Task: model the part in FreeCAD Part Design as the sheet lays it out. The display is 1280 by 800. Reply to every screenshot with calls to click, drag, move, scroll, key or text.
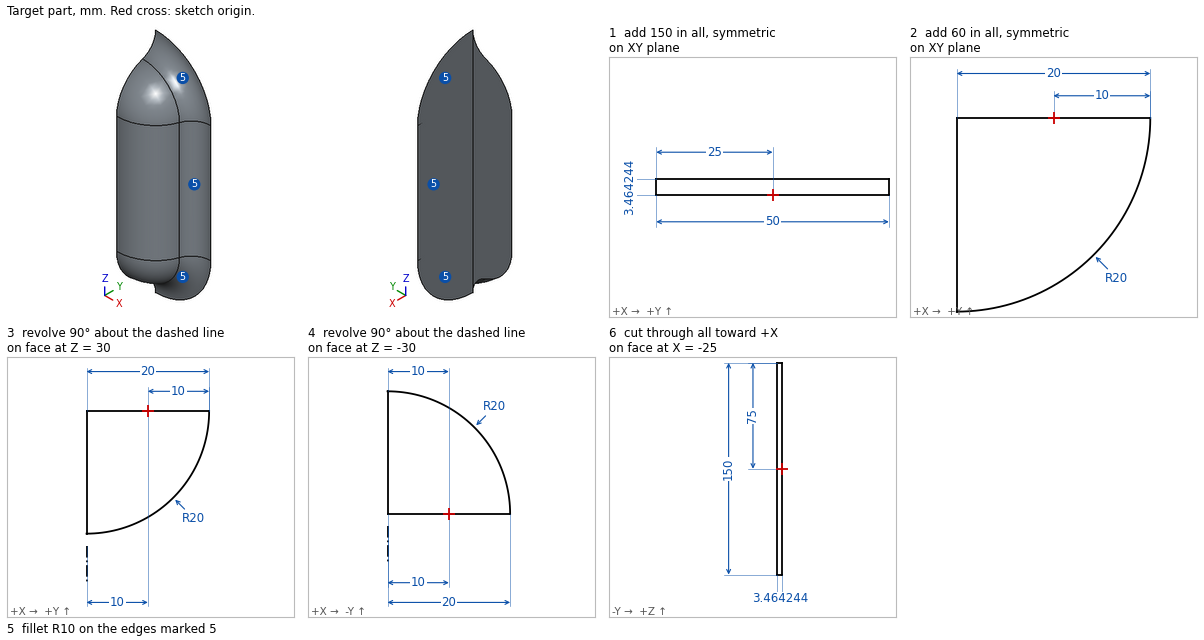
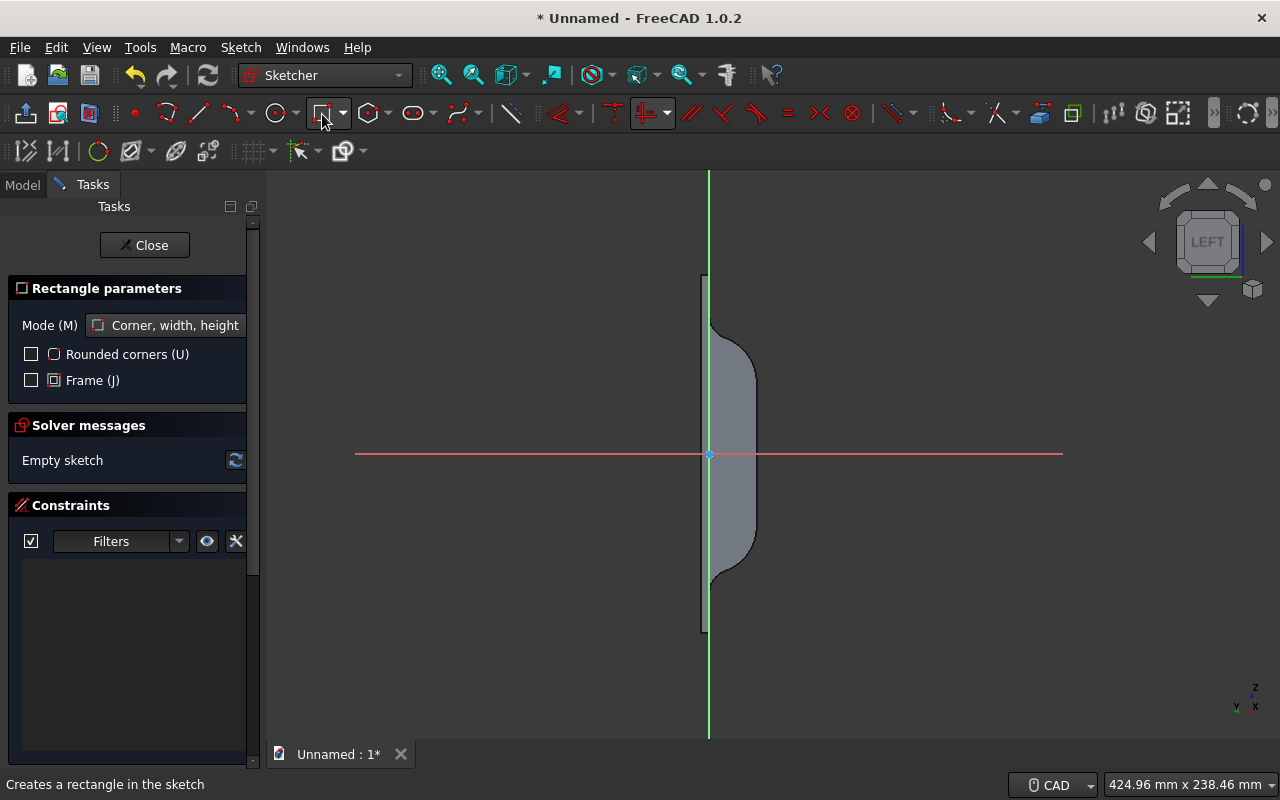
scroll(701, 275, up, 4)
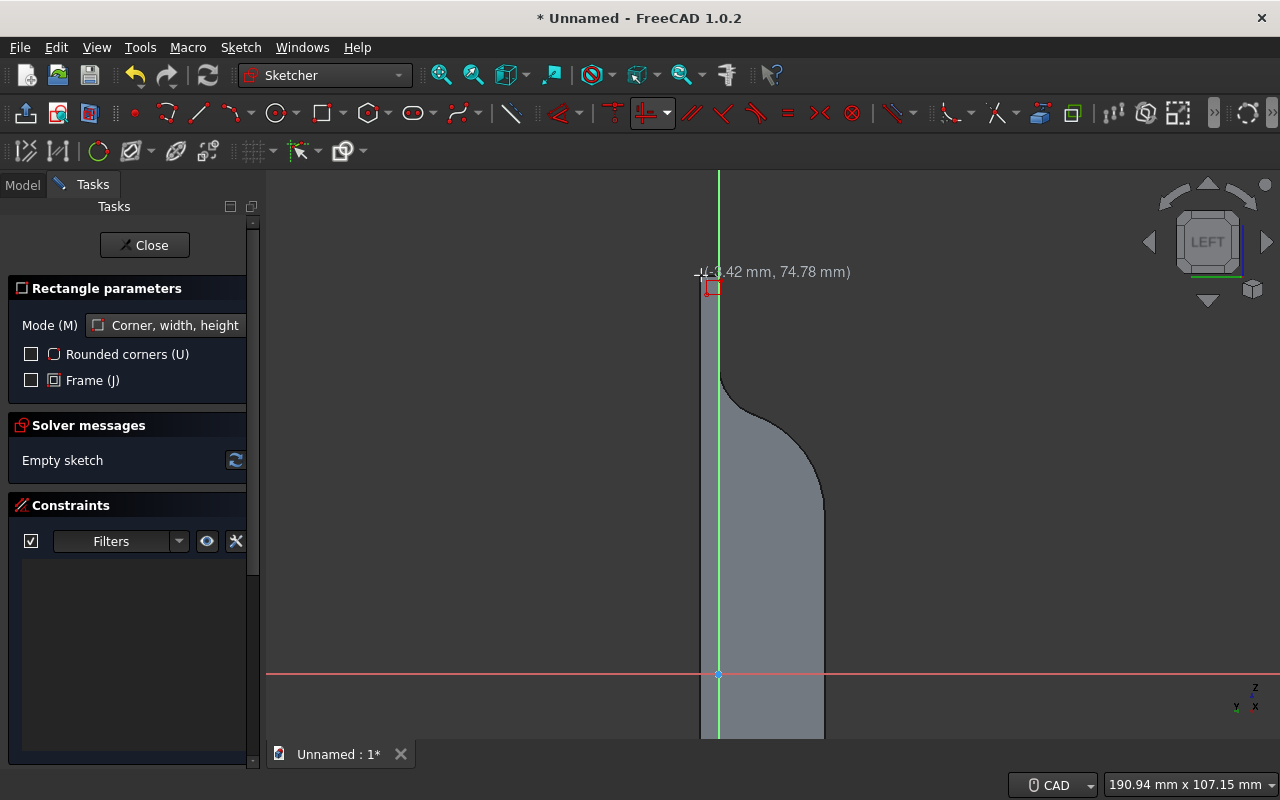
click(700, 276)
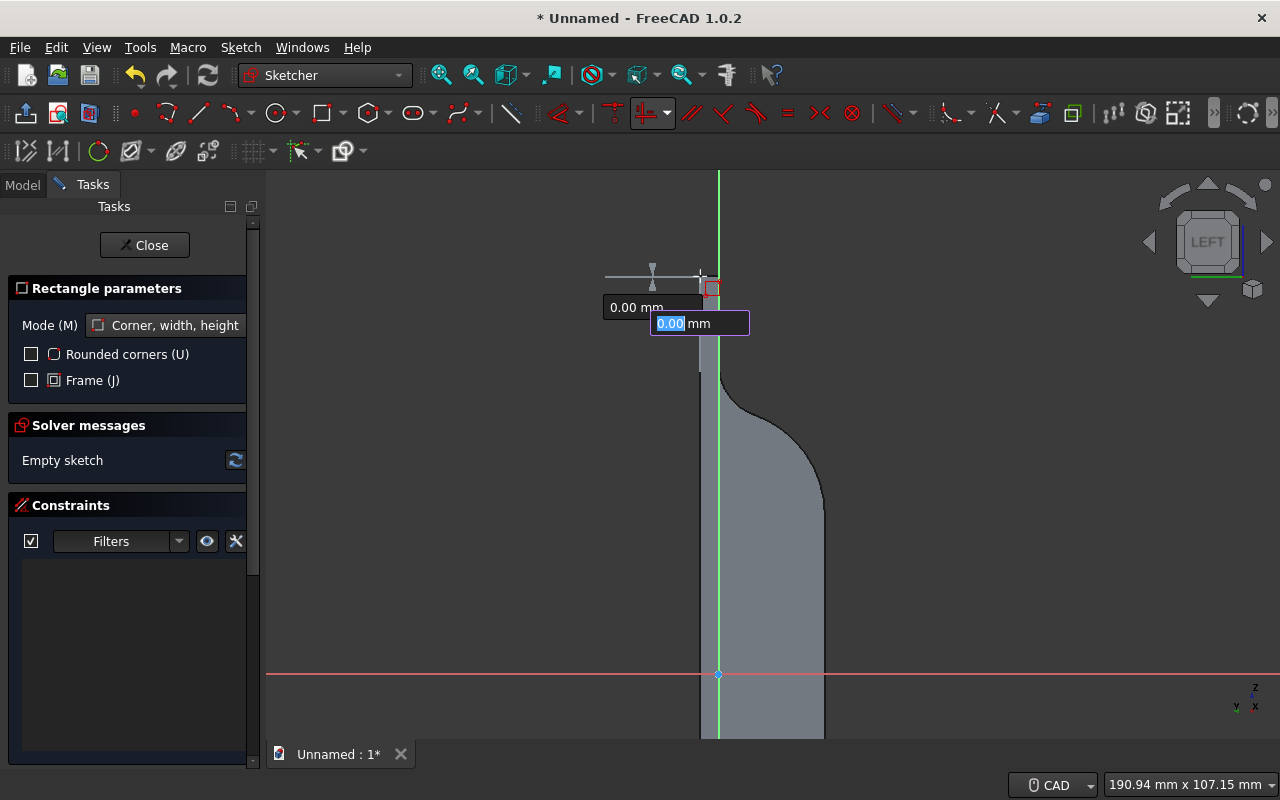
scroll(700, 275, down, 4)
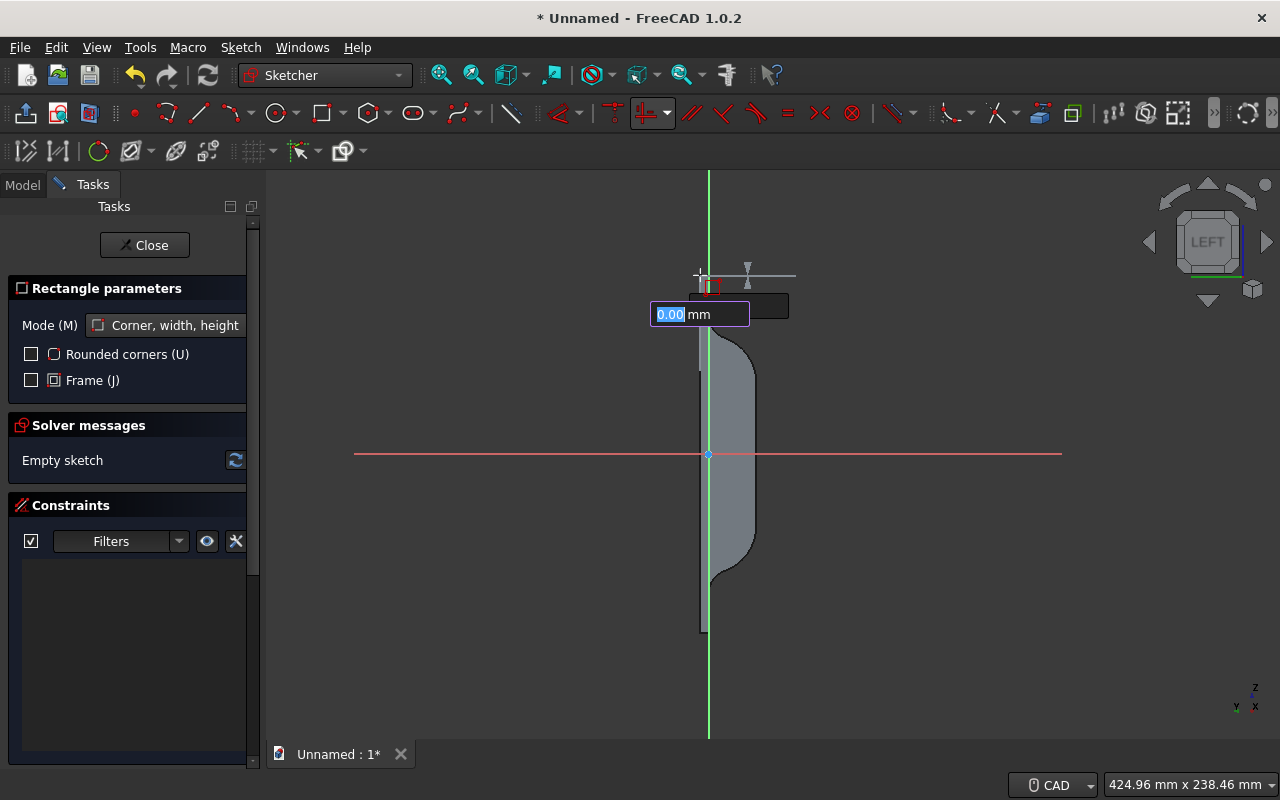
click(709, 633)
key(Escape)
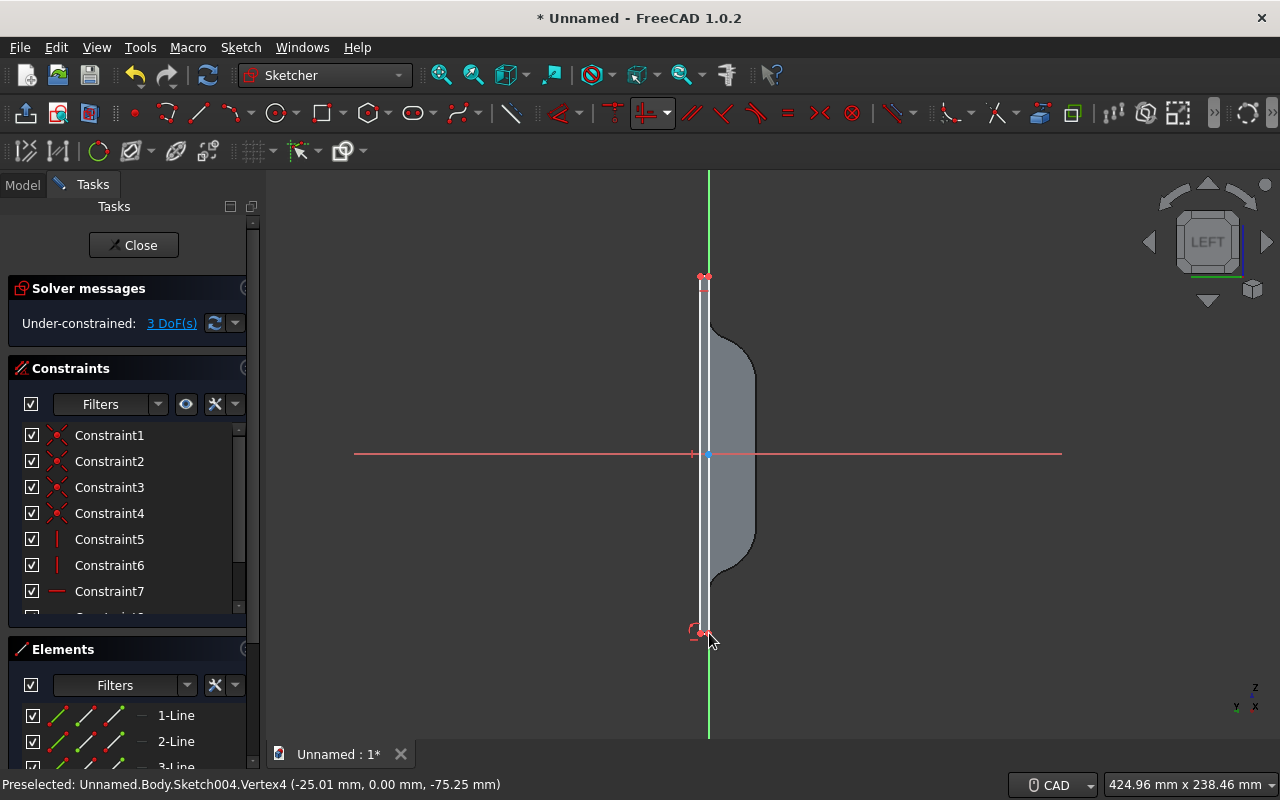
click(558, 114)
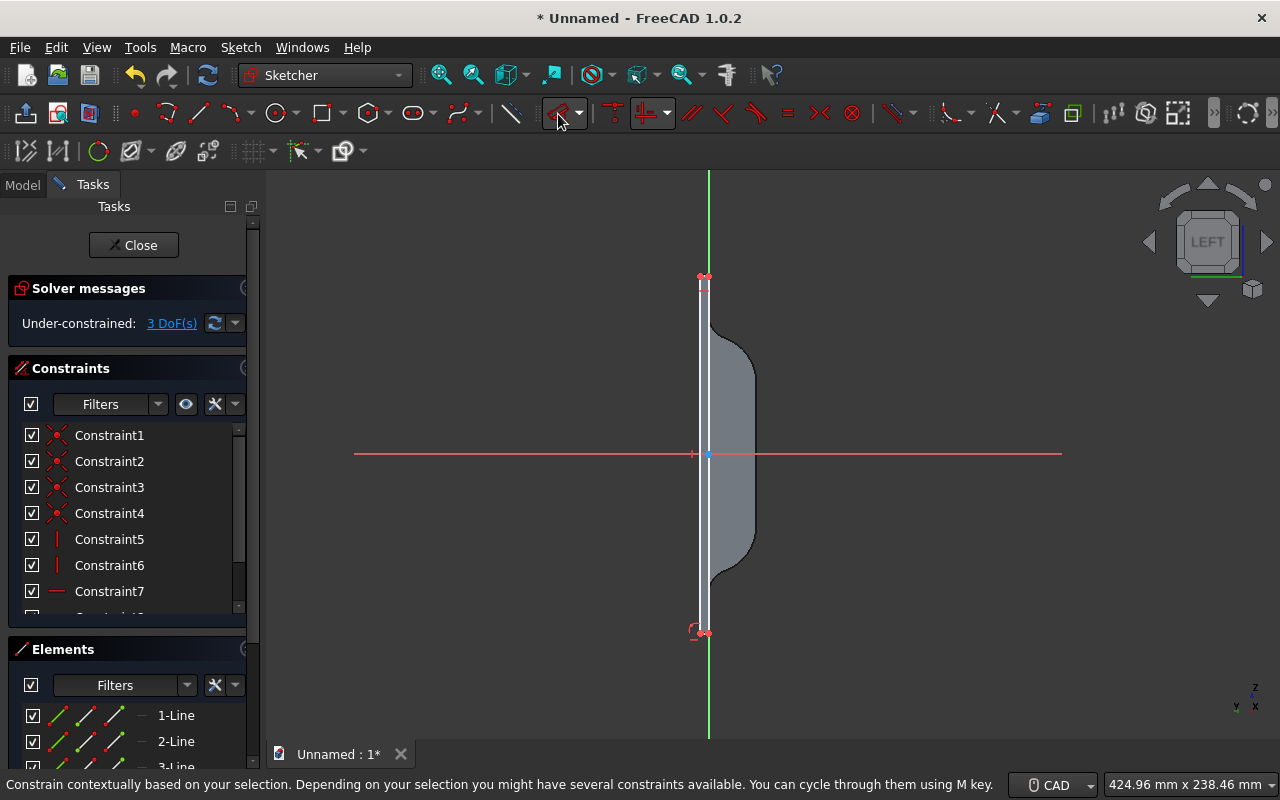
scroll(700, 383, up, 3)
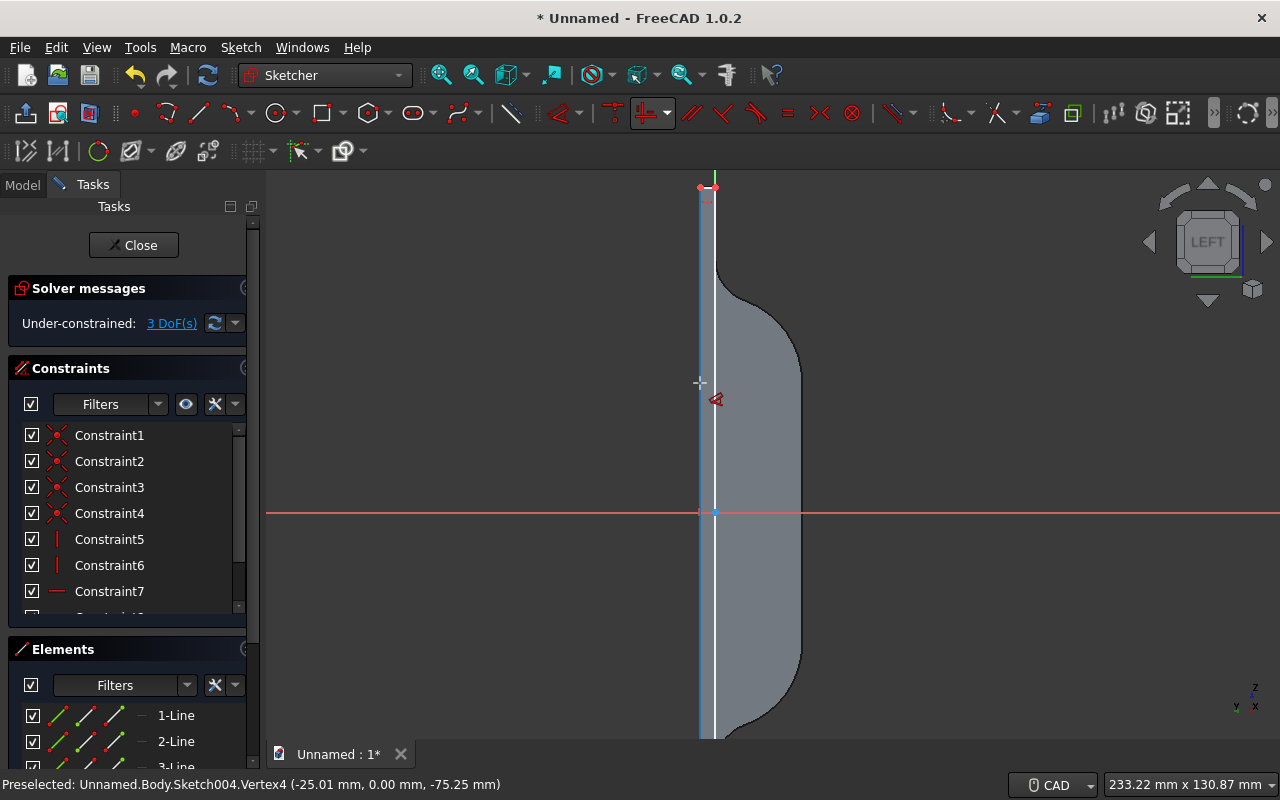
click(700, 383)
click(666, 454)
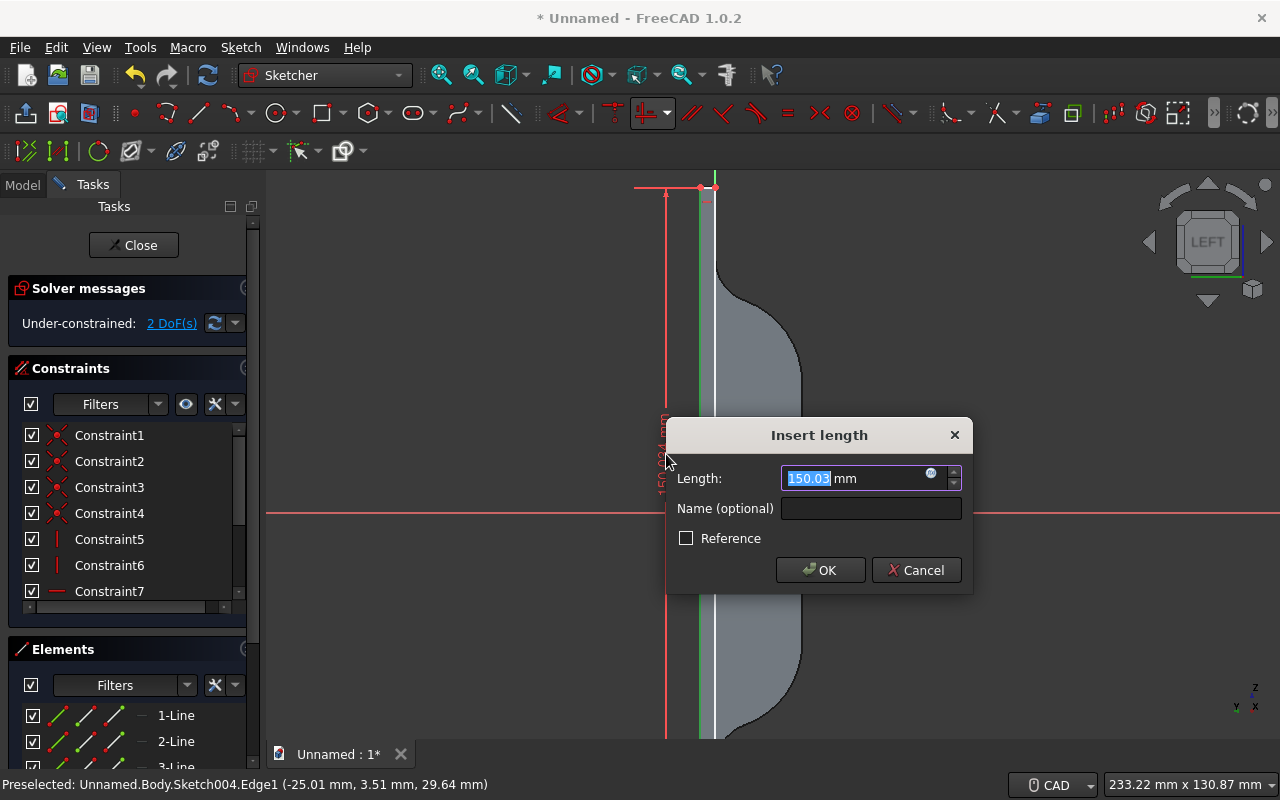
text(150)
key(Return)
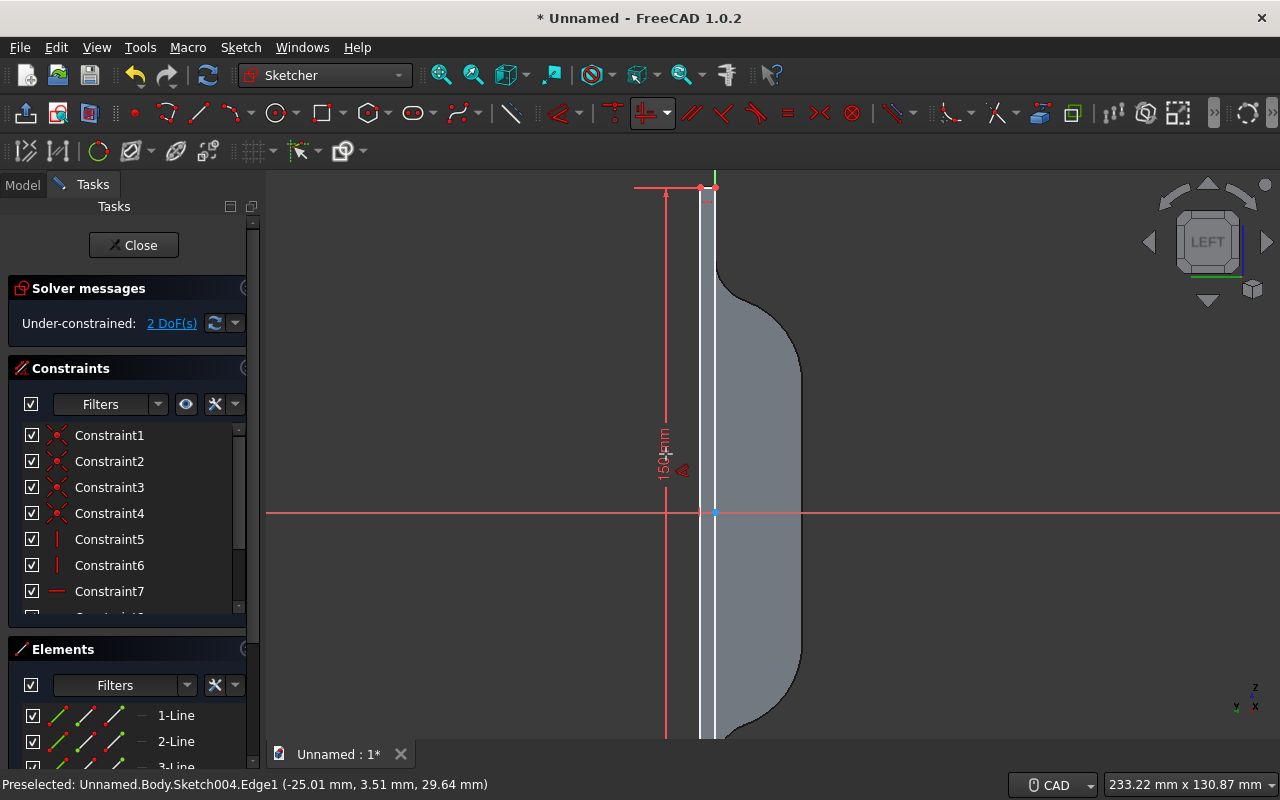
scroll(700, 383, down, 3)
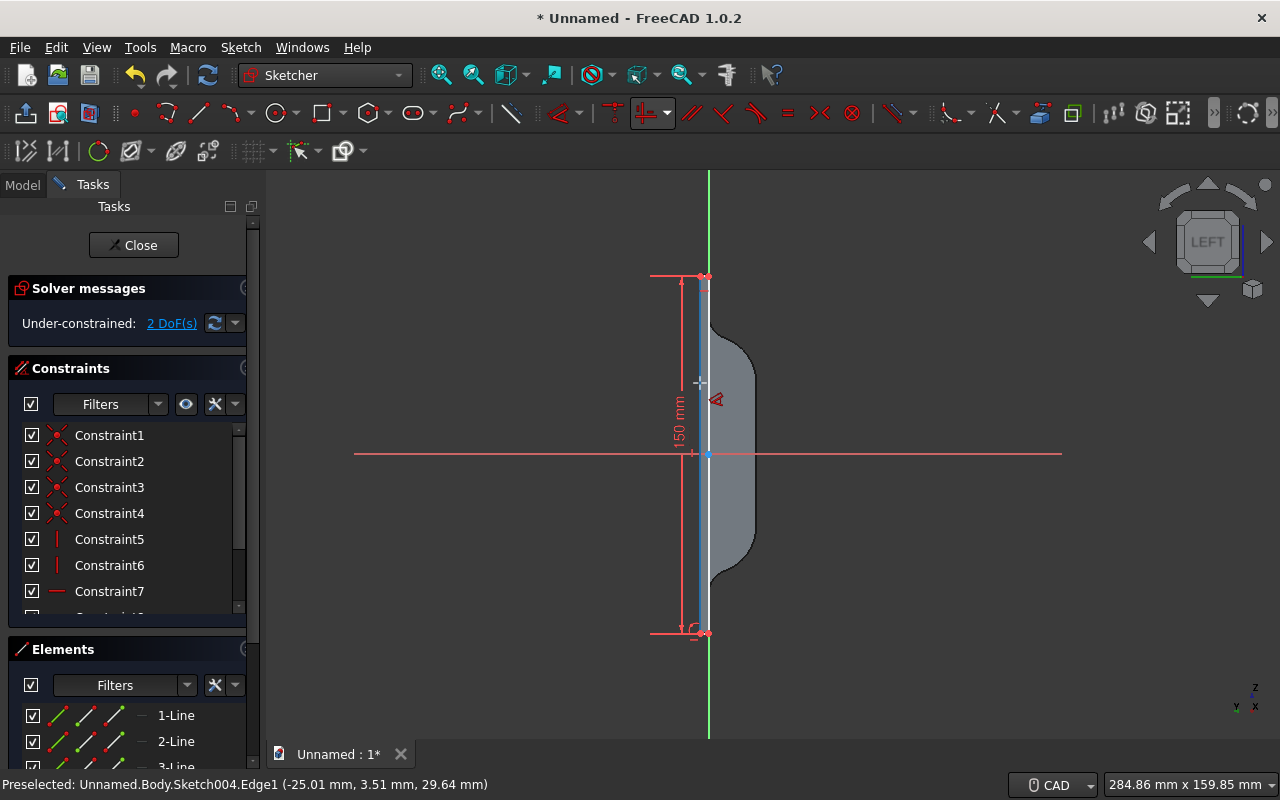
scroll(700, 276, up, 2)